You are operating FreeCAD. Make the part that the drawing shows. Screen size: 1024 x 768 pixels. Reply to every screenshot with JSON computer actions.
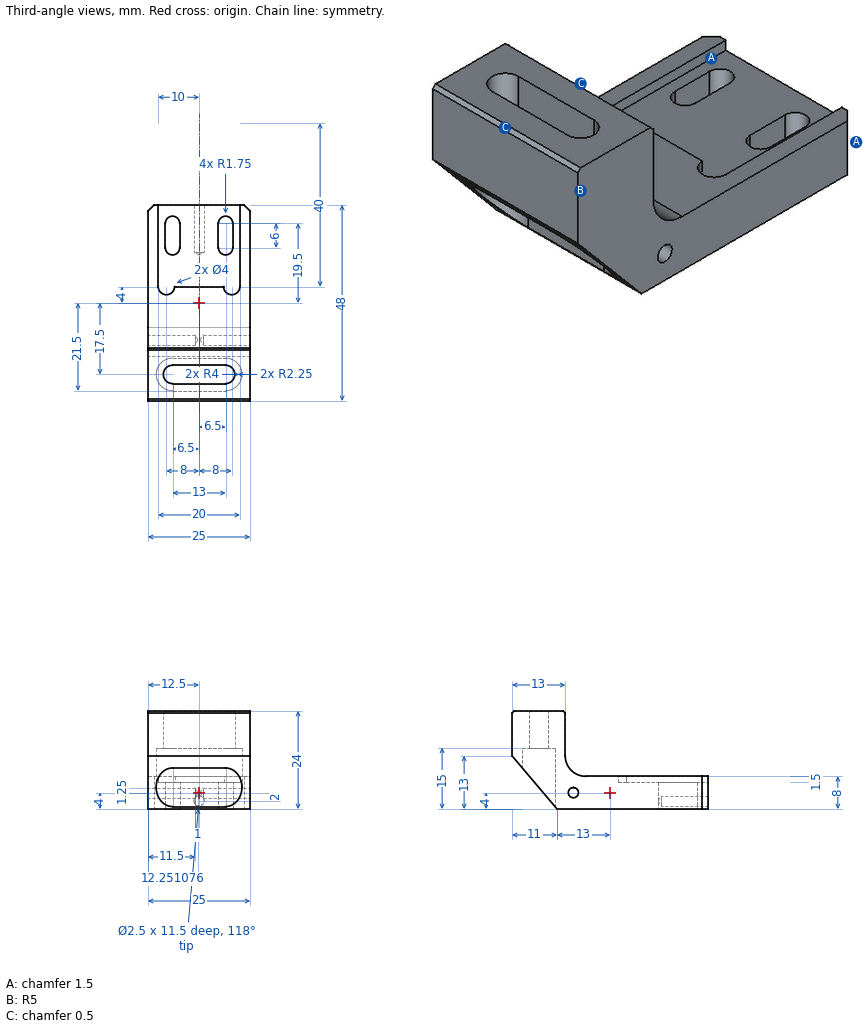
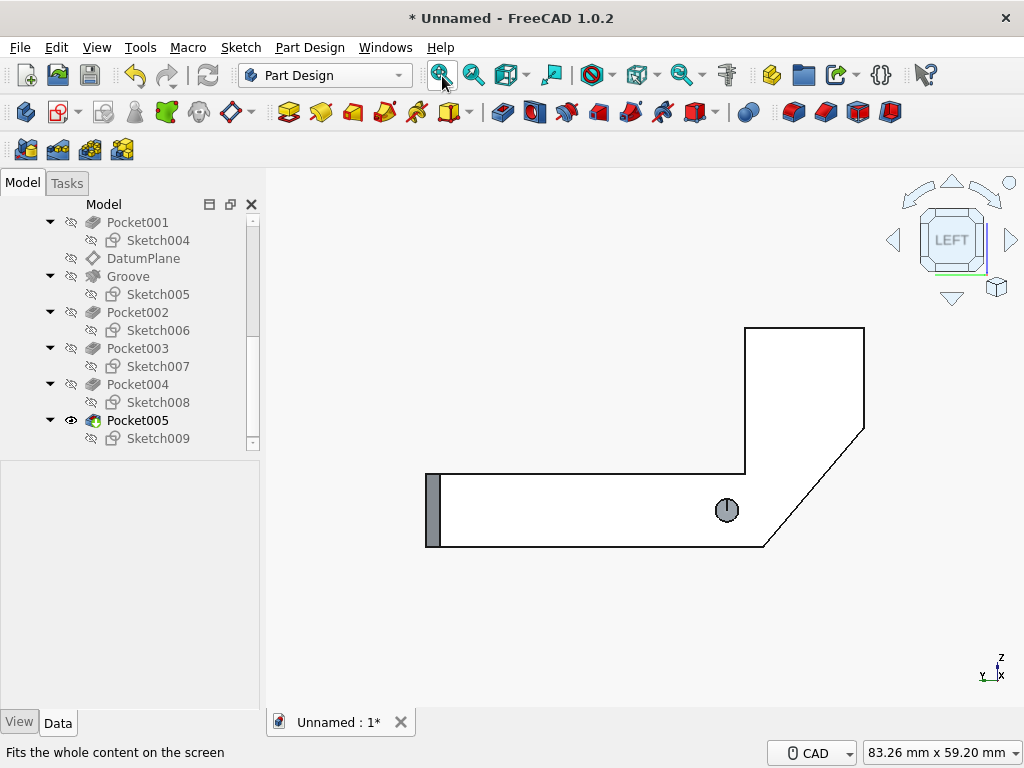
{"action": "key", "text": "v 3"}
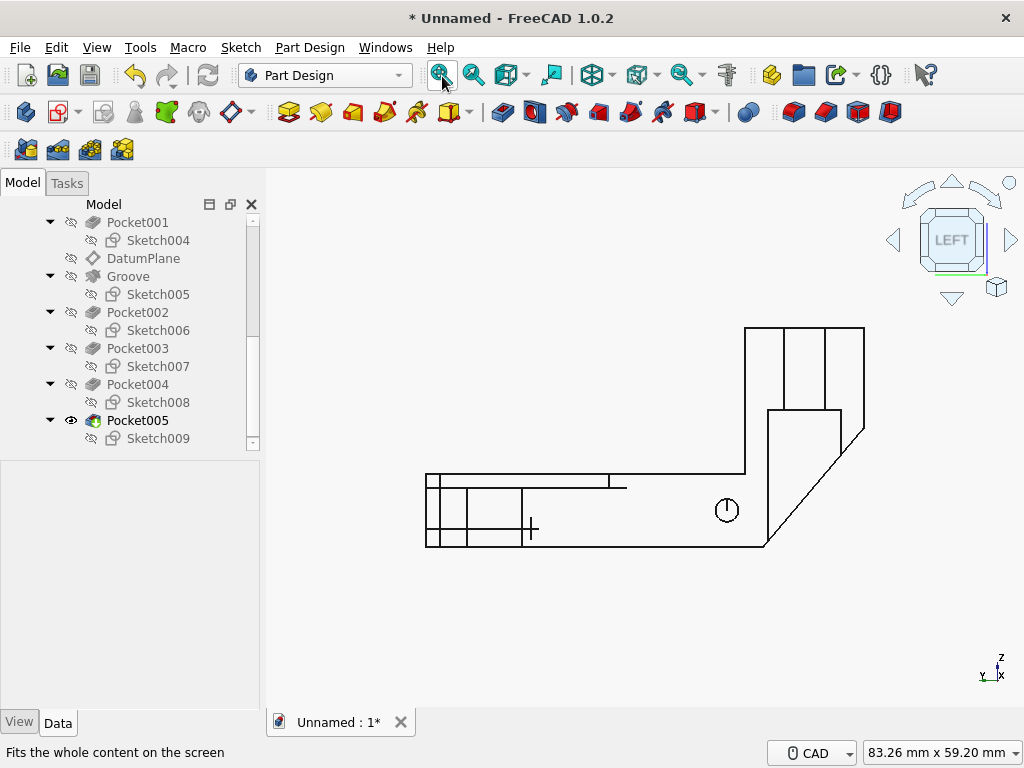
{"action": "key", "text": "0"}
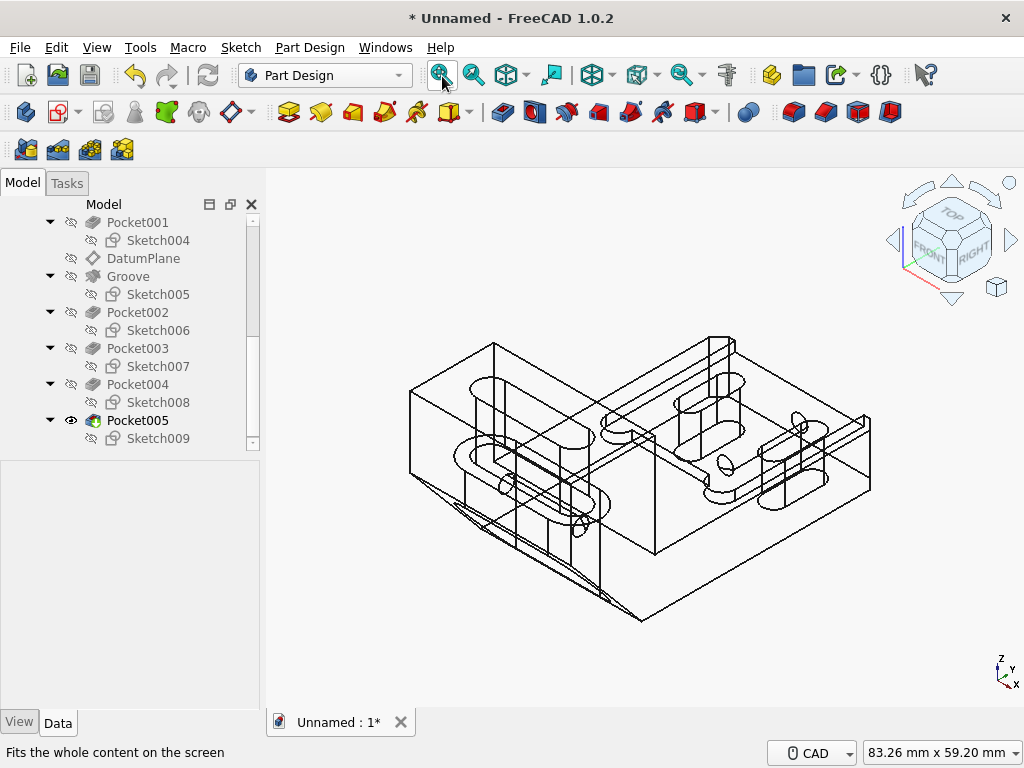
{"action": "left_click", "coordinate": [606, 526]}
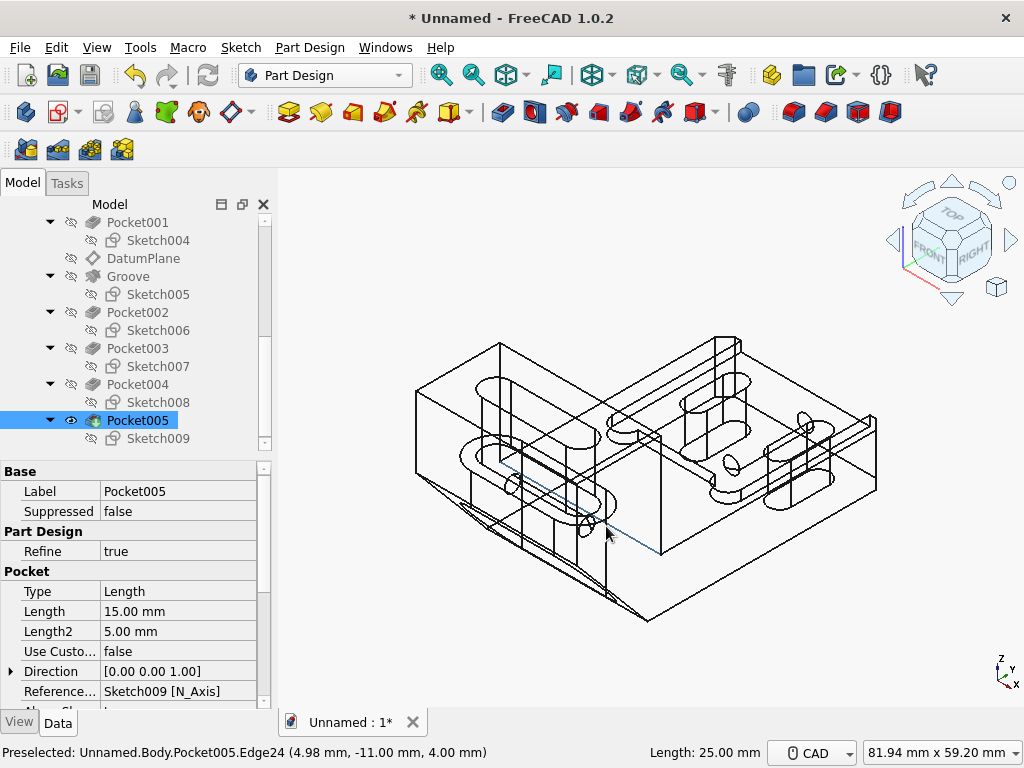
{"action": "key", "text": "v 1"}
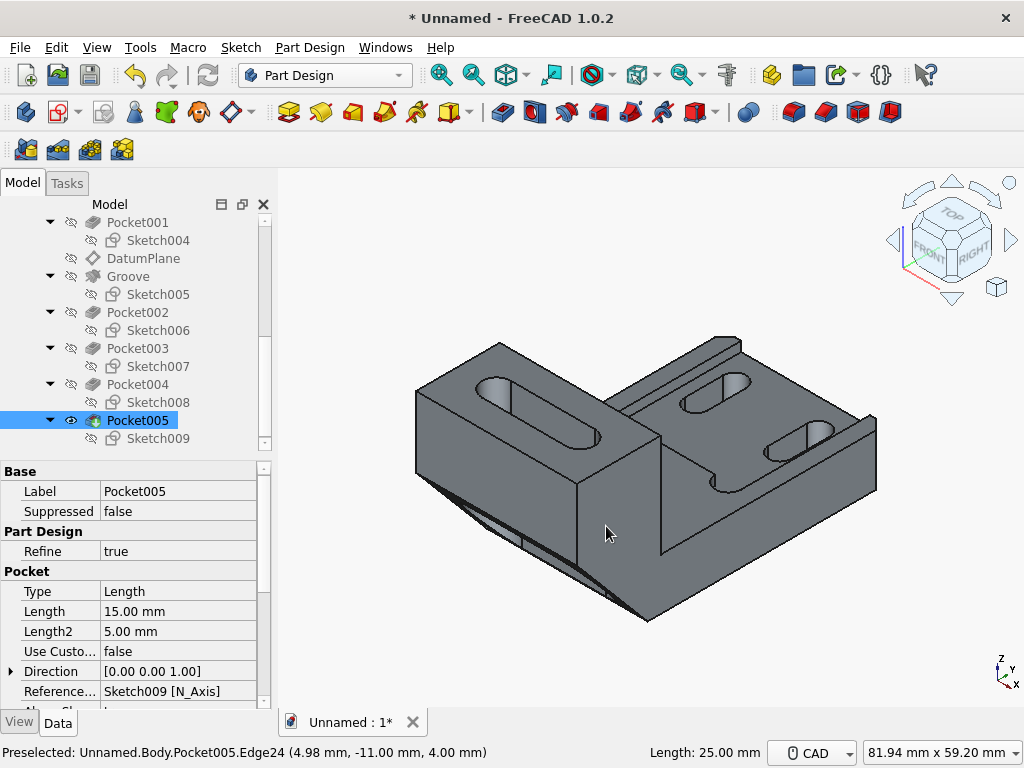
{"action": "left_click", "coordinate": [794, 112]}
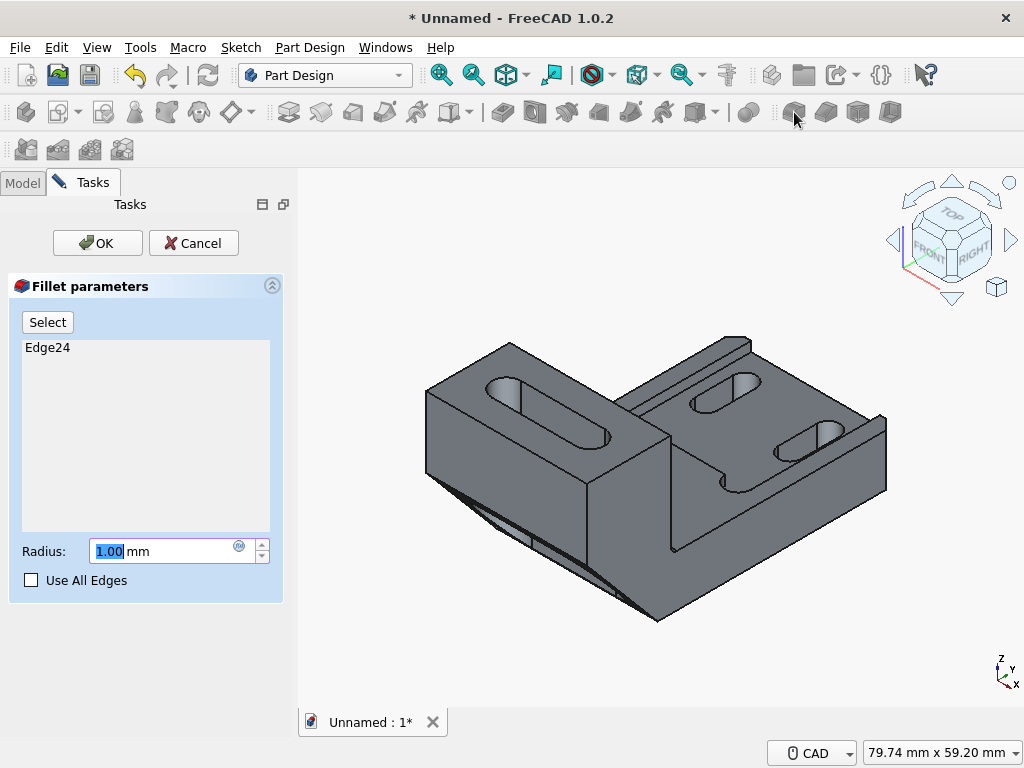
{"action": "type", "text": "5"}
{"action": "key", "text": "Tab"}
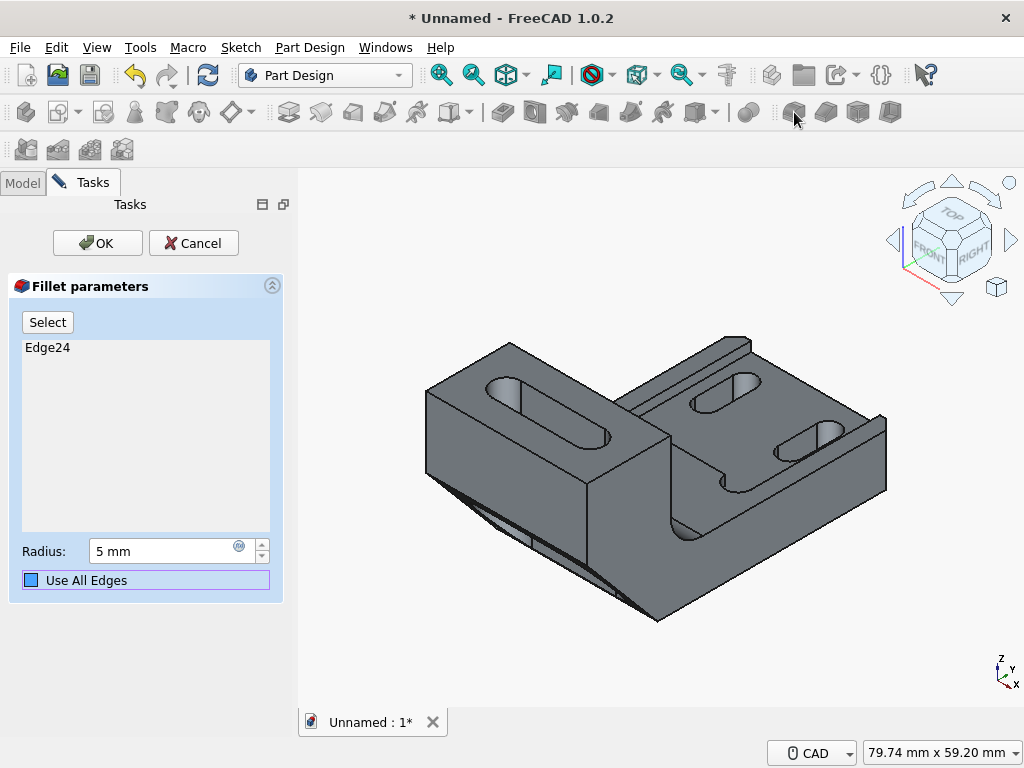
{"action": "left_click", "coordinate": [98, 243]}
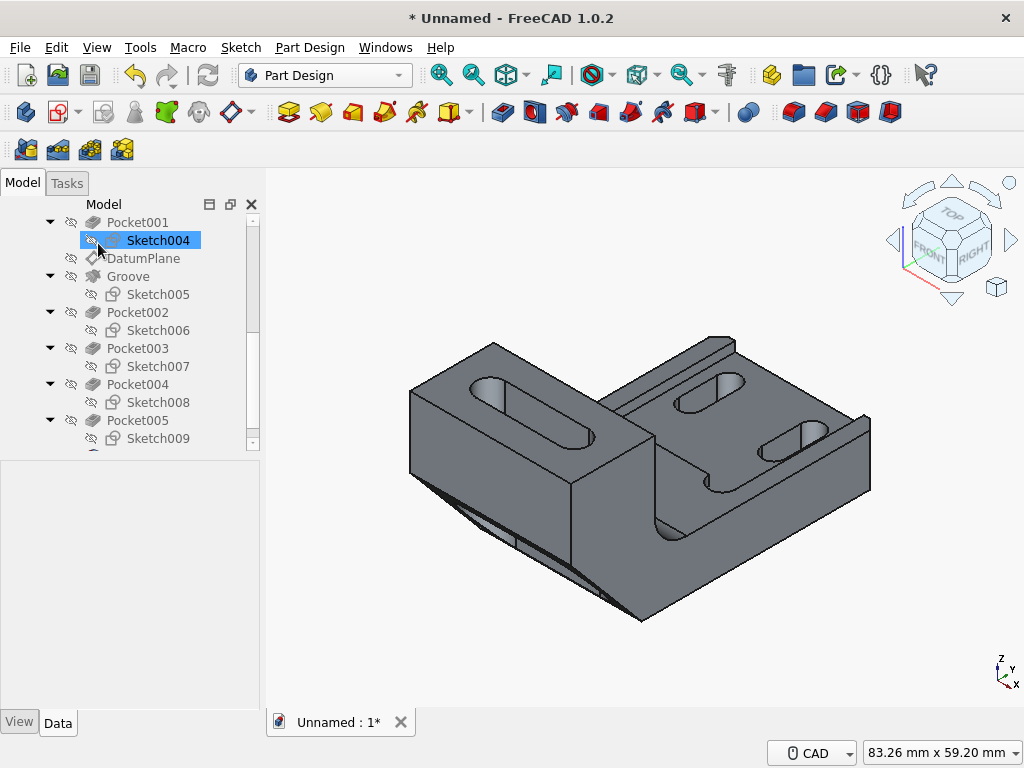
{"action": "left_click", "coordinate": [116, 276]}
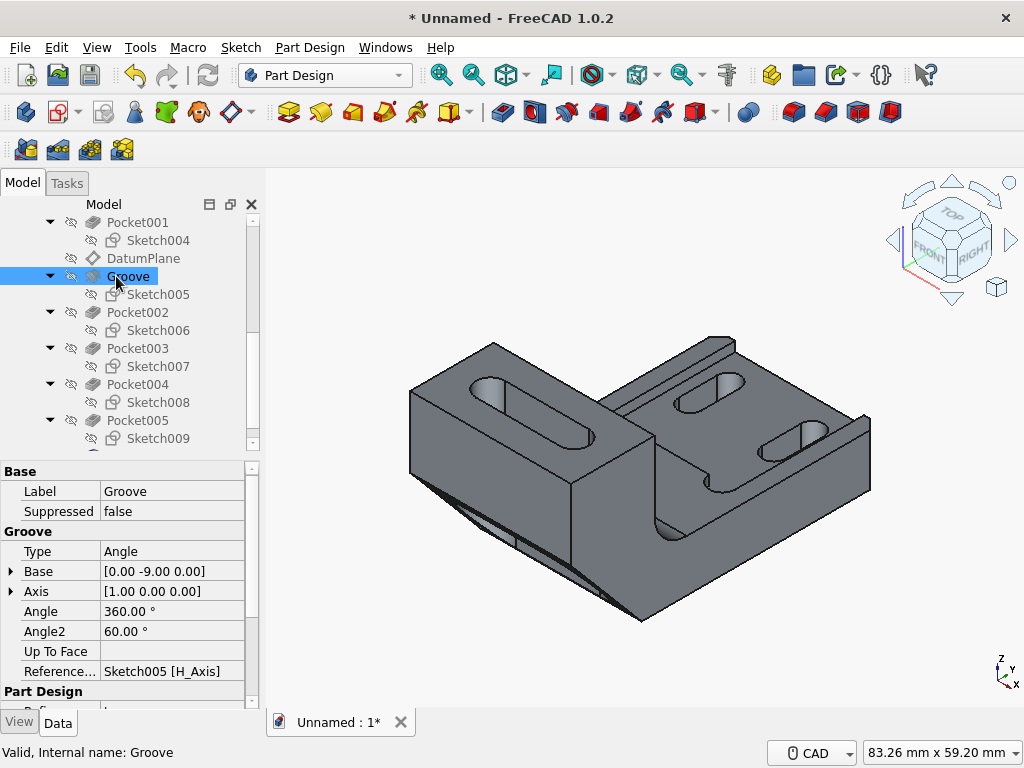
{"action": "left_click", "coordinate": [26, 150]}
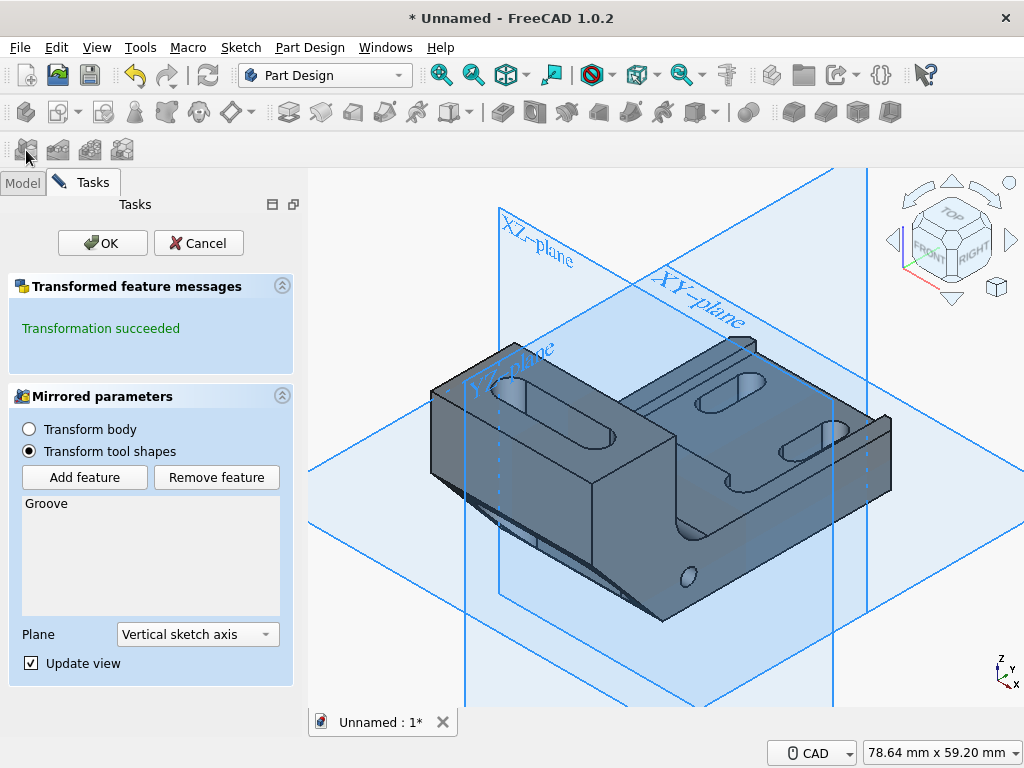
{"action": "left_click", "coordinate": [198, 634]}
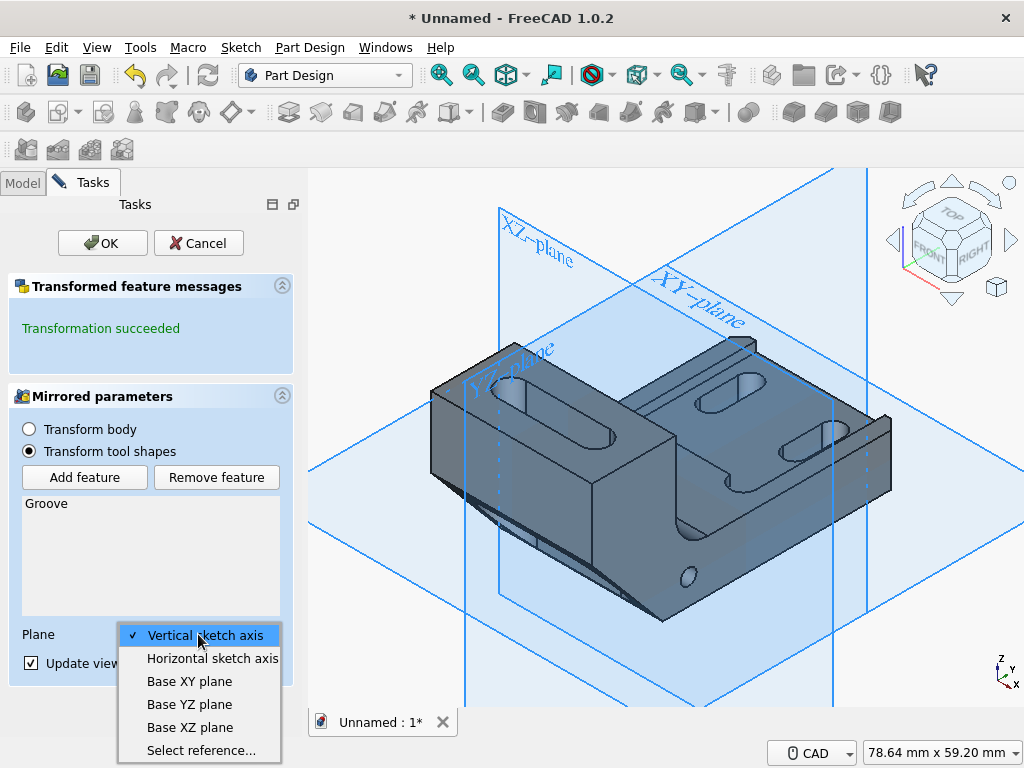
{"action": "left_click", "coordinate": [198, 704]}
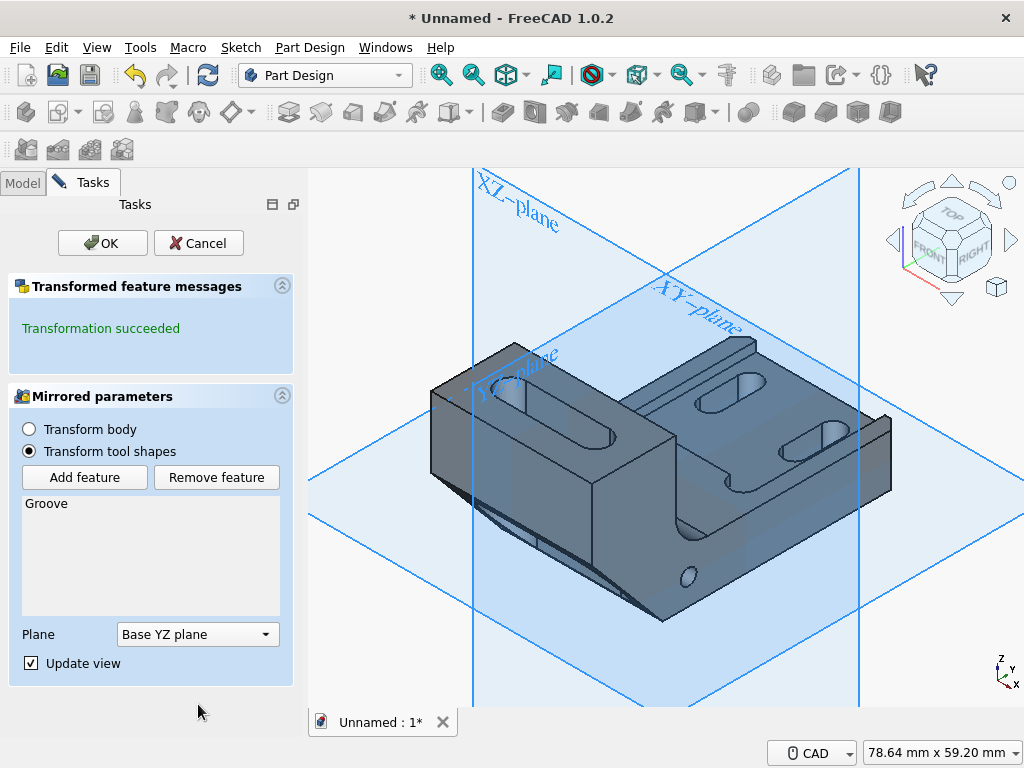
{"action": "left_click", "coordinate": [103, 243]}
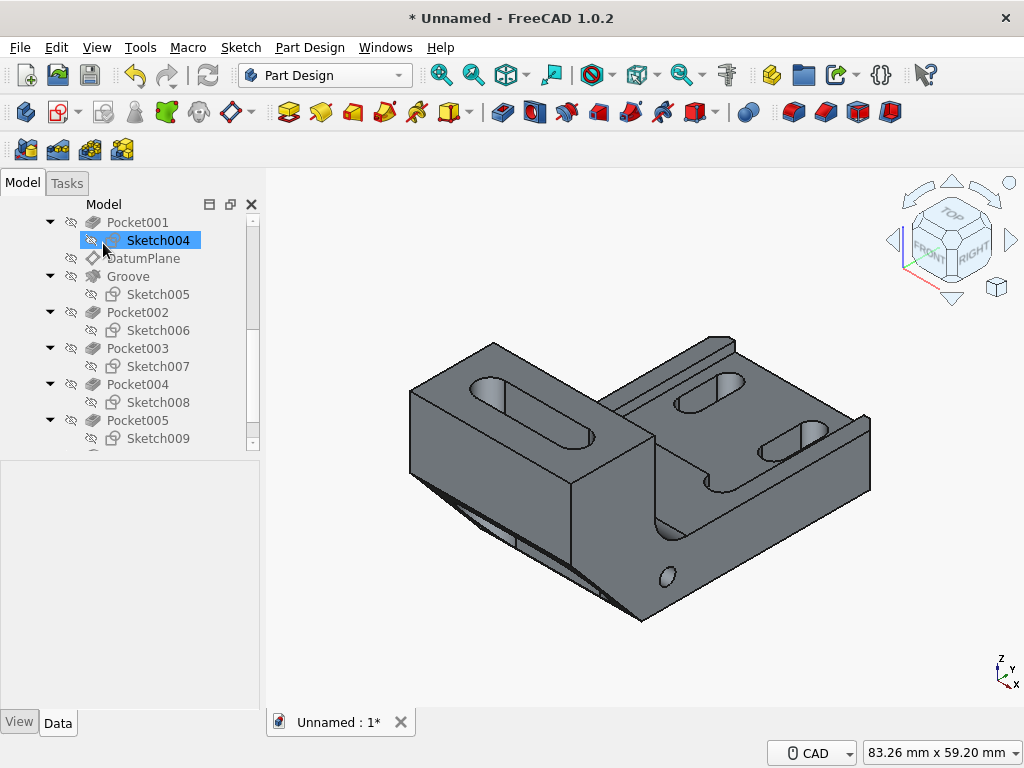
{"action": "left_click", "coordinate": [490, 437]}